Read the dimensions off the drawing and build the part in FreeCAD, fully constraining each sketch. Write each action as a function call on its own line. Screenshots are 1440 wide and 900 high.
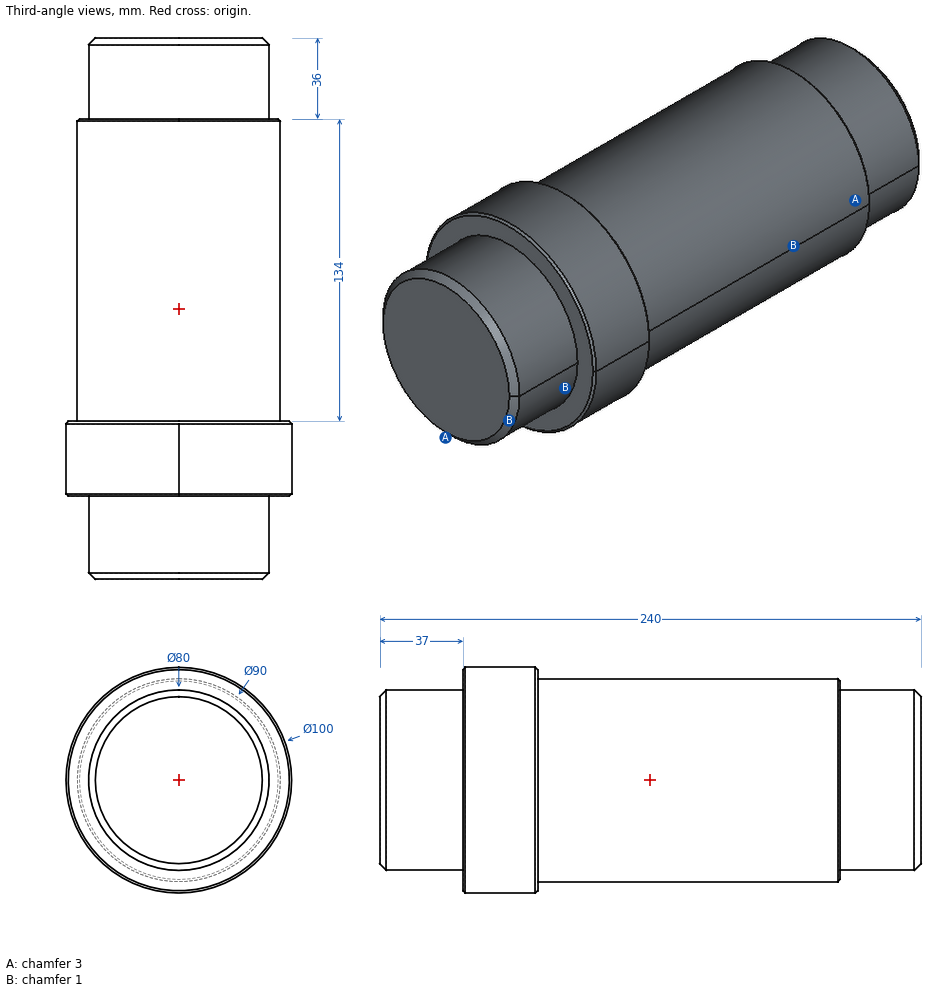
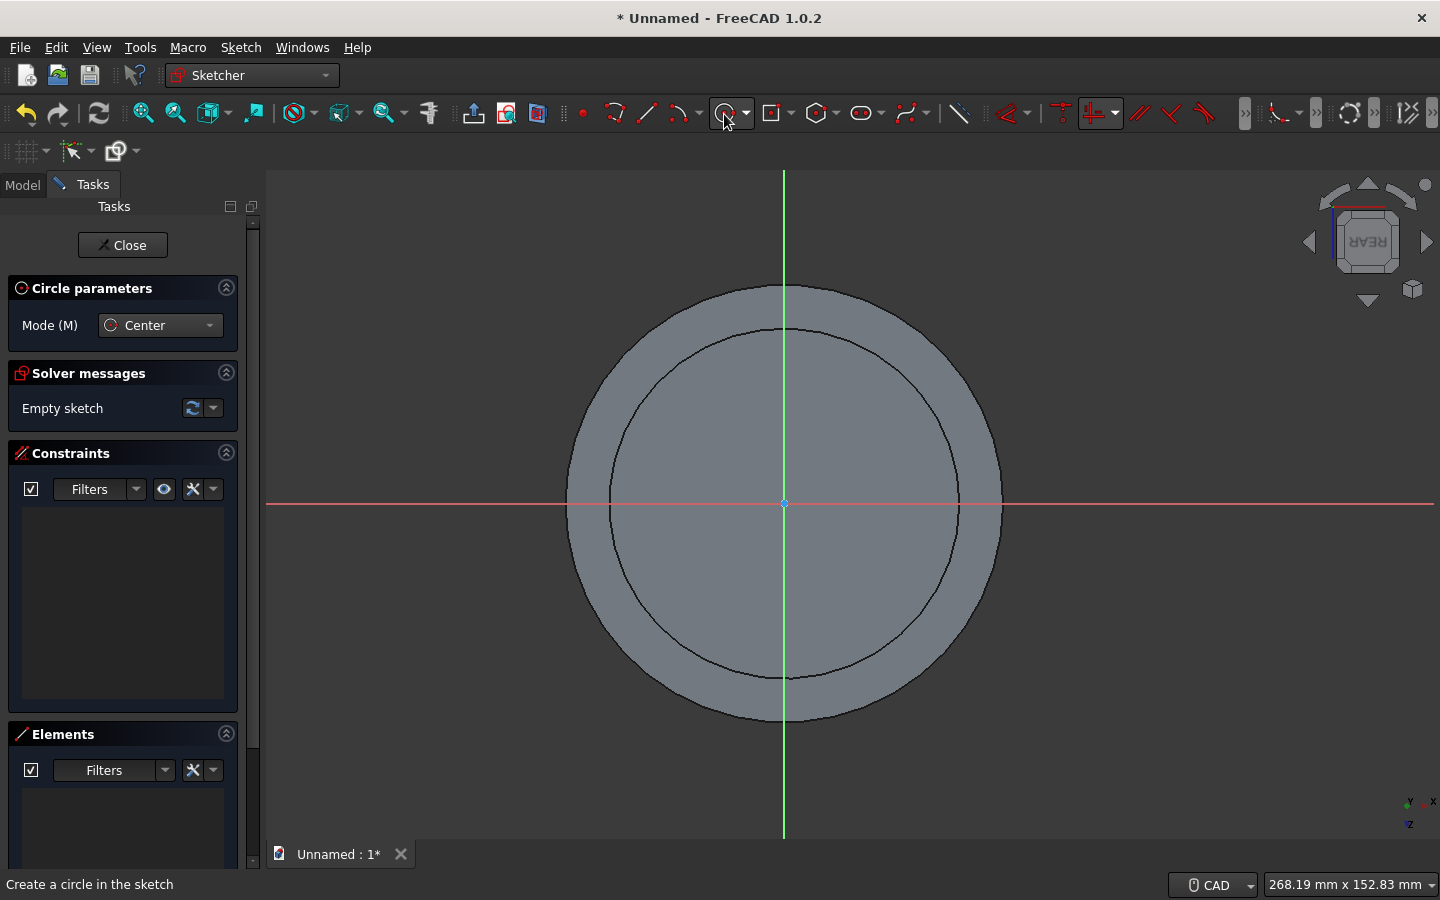
click(784, 504)
click(939, 349)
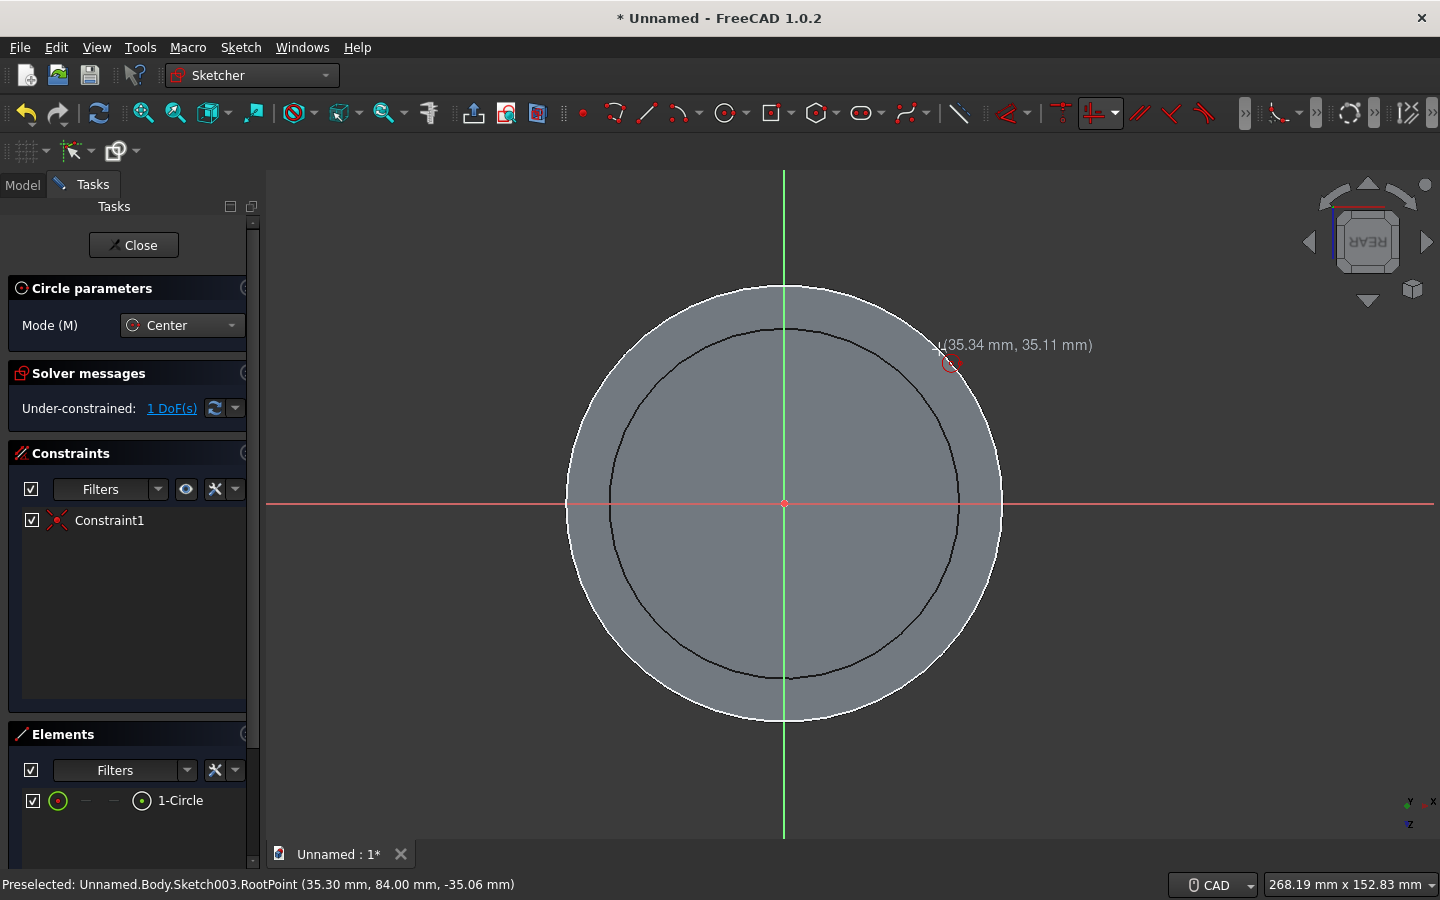
click(784, 504)
click(924, 364)
key(Escape)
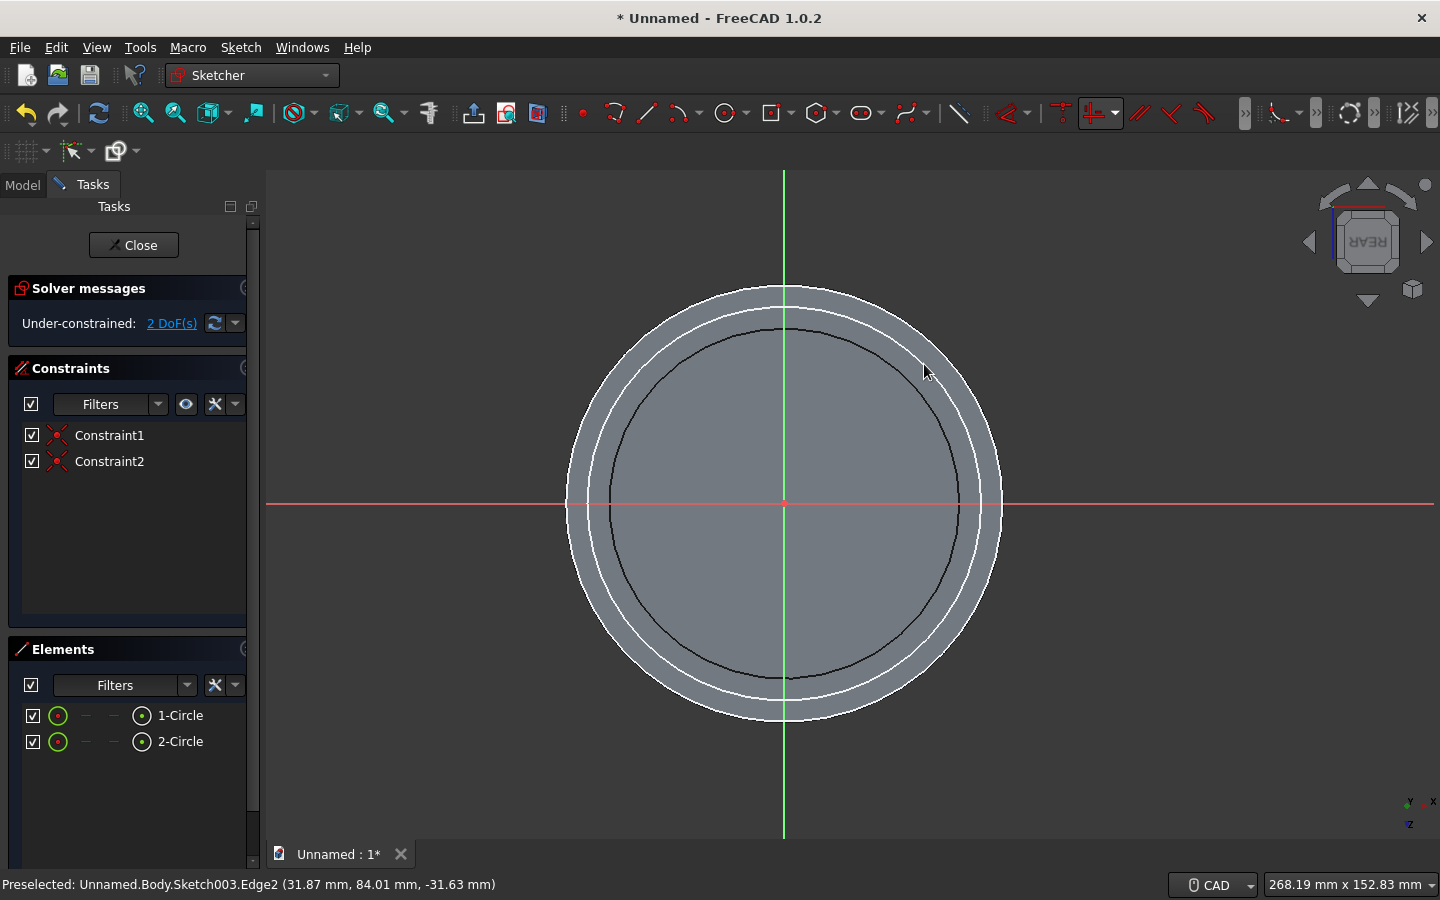
click(1006, 114)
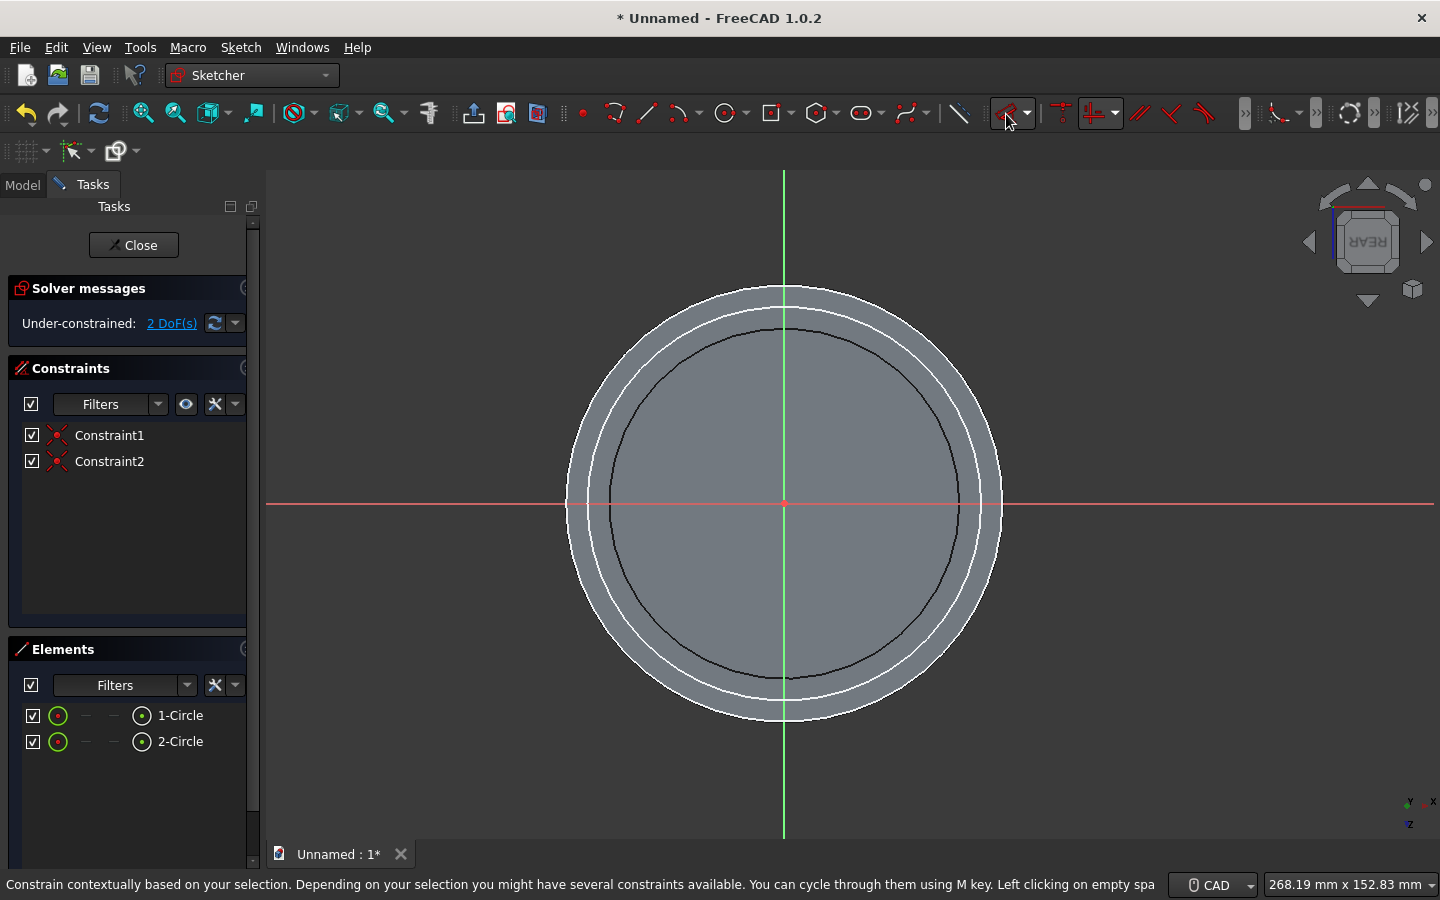
click(938, 349)
click(961, 326)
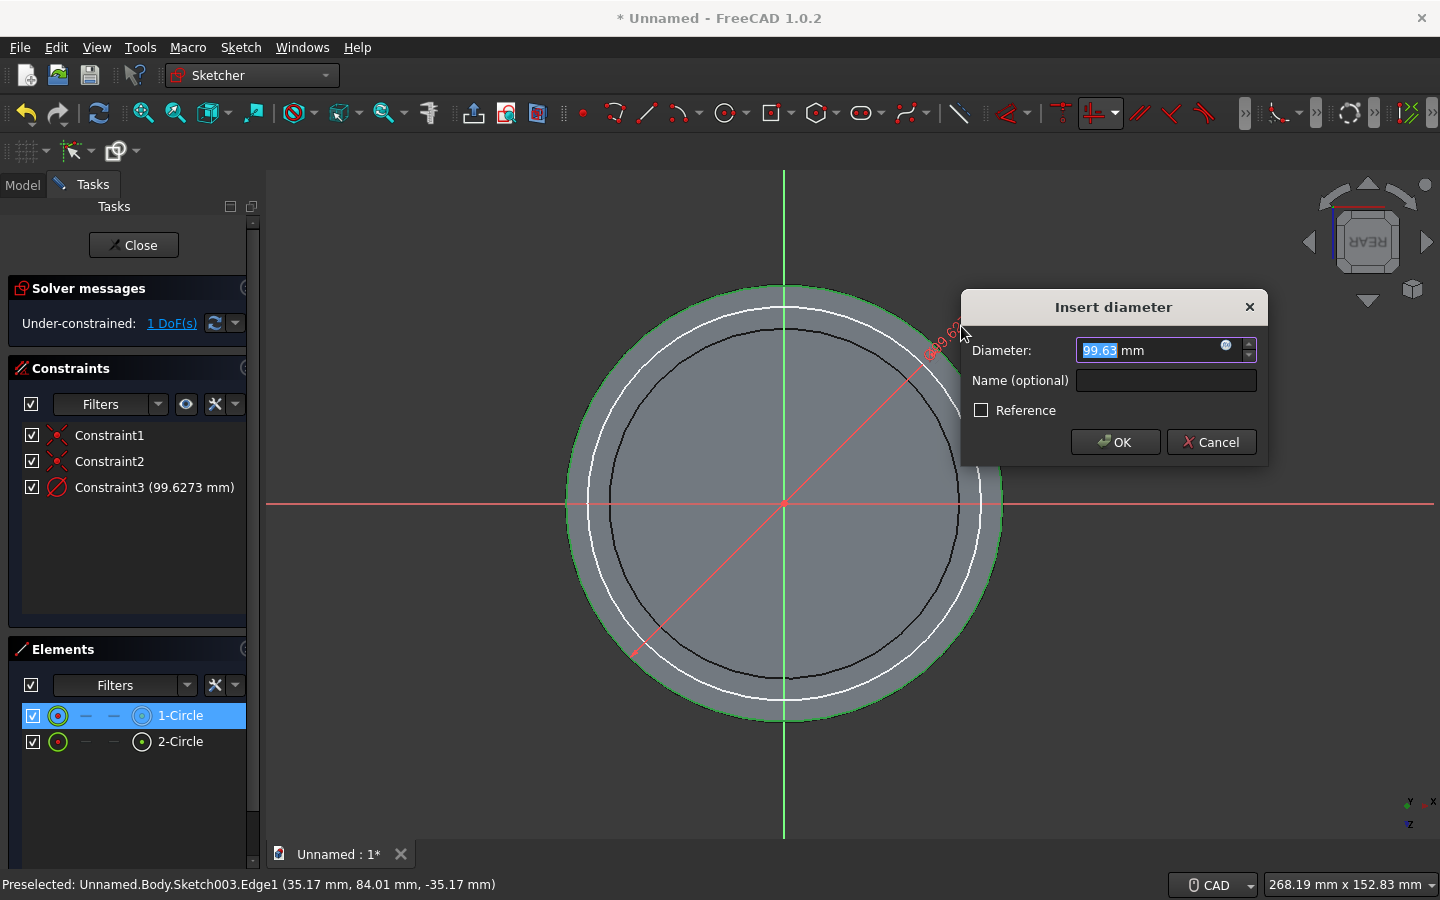
text(100)
key(Return)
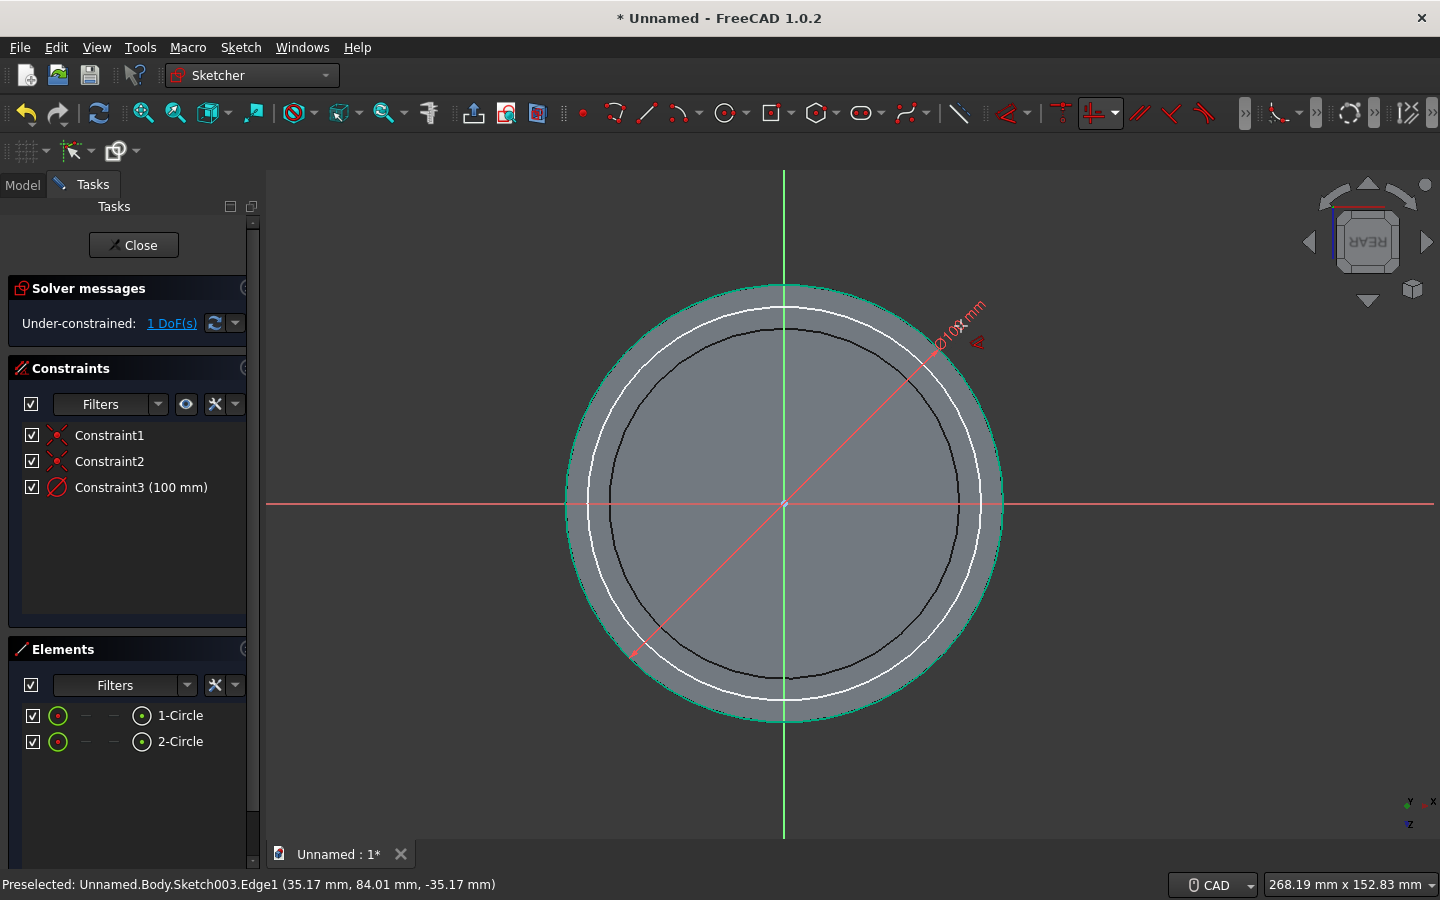
click(923, 364)
click(1026, 432)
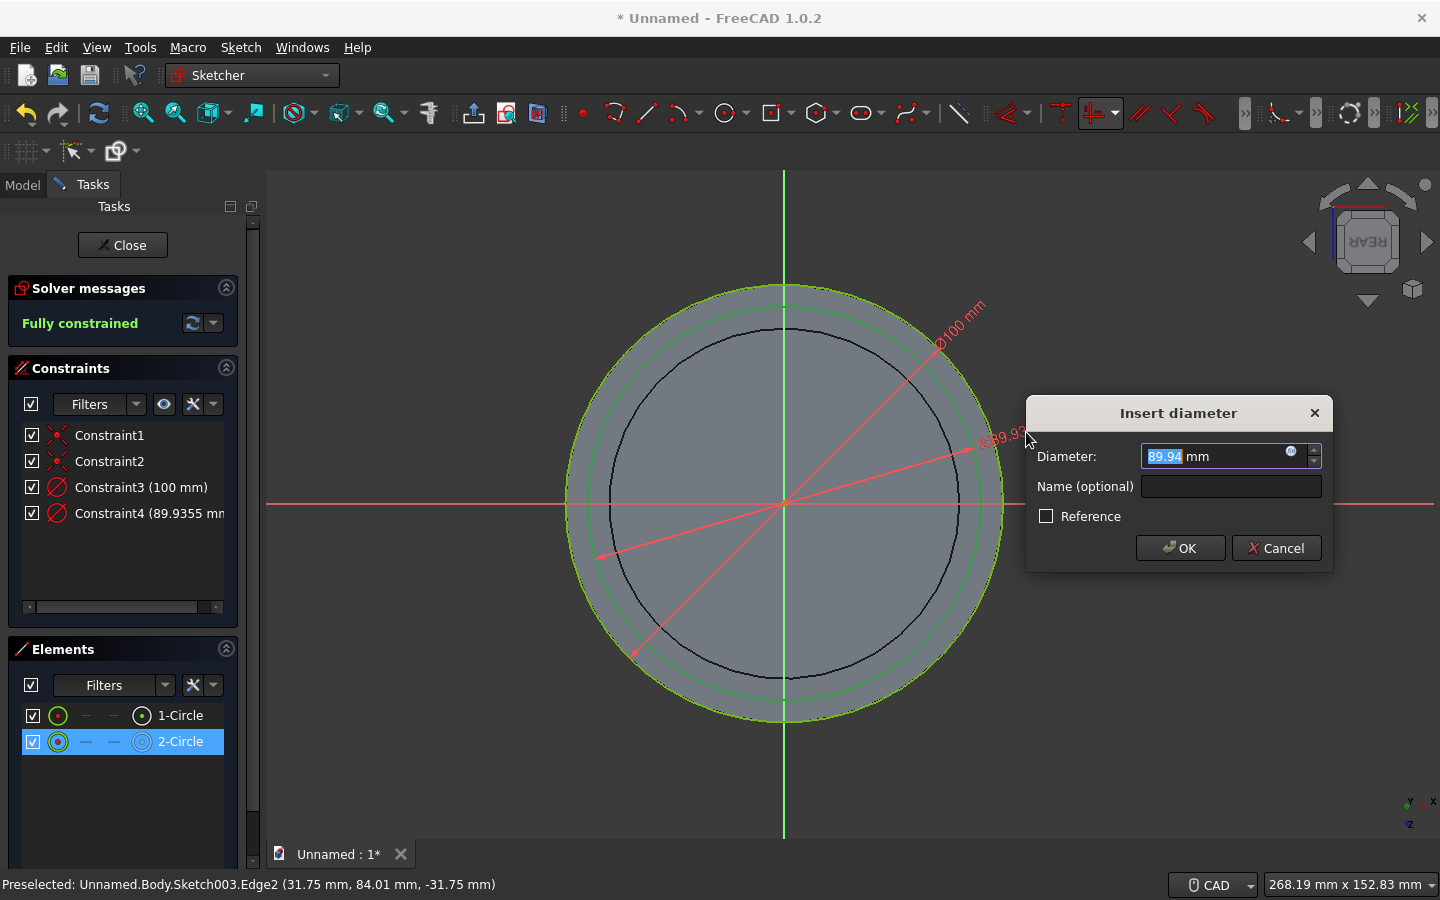
text(90)
key(Return)
key(Escape)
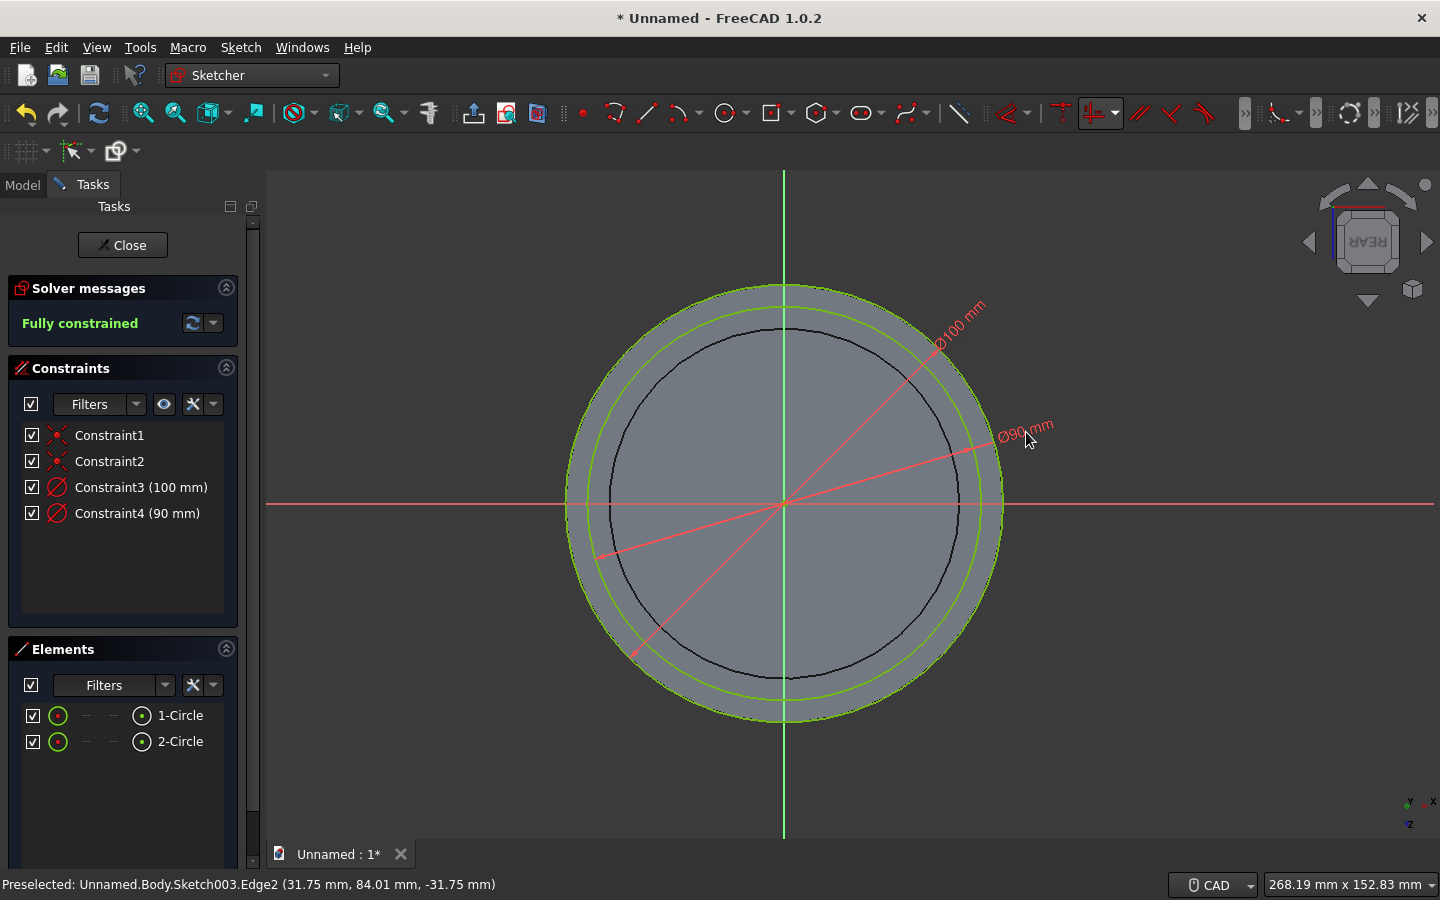
click(123, 245)